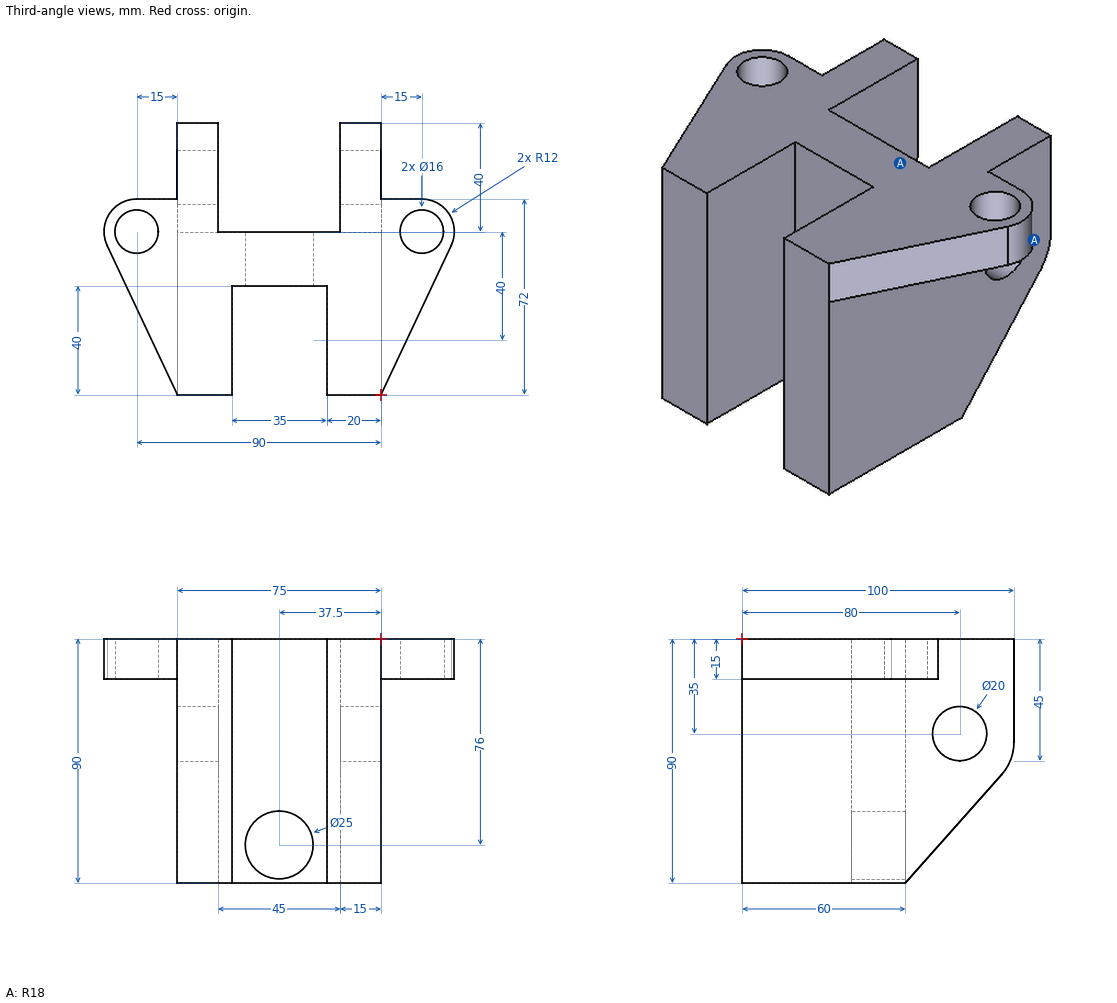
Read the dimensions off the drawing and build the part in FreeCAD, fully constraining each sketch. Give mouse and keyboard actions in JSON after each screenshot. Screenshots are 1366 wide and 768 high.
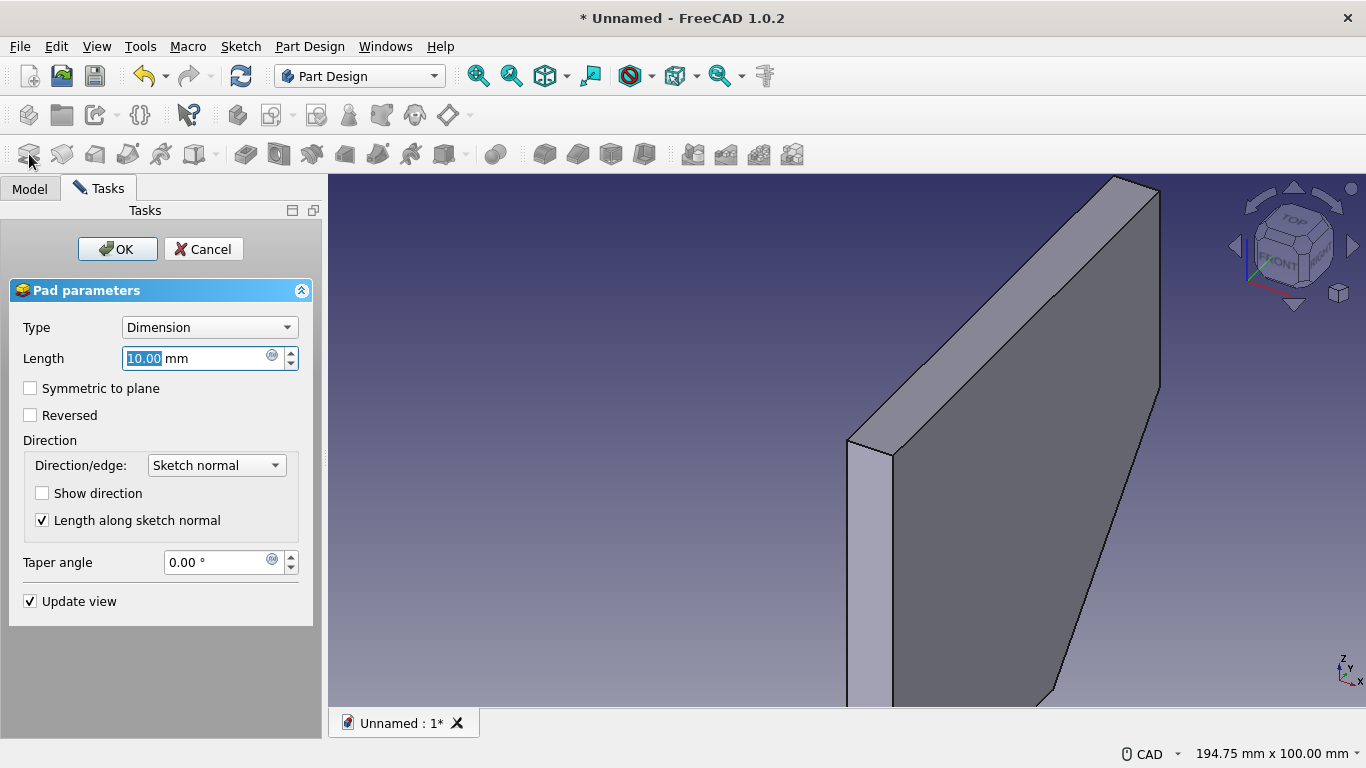
{"action": "type", "text": "75"}
{"action": "key", "text": "Tab"}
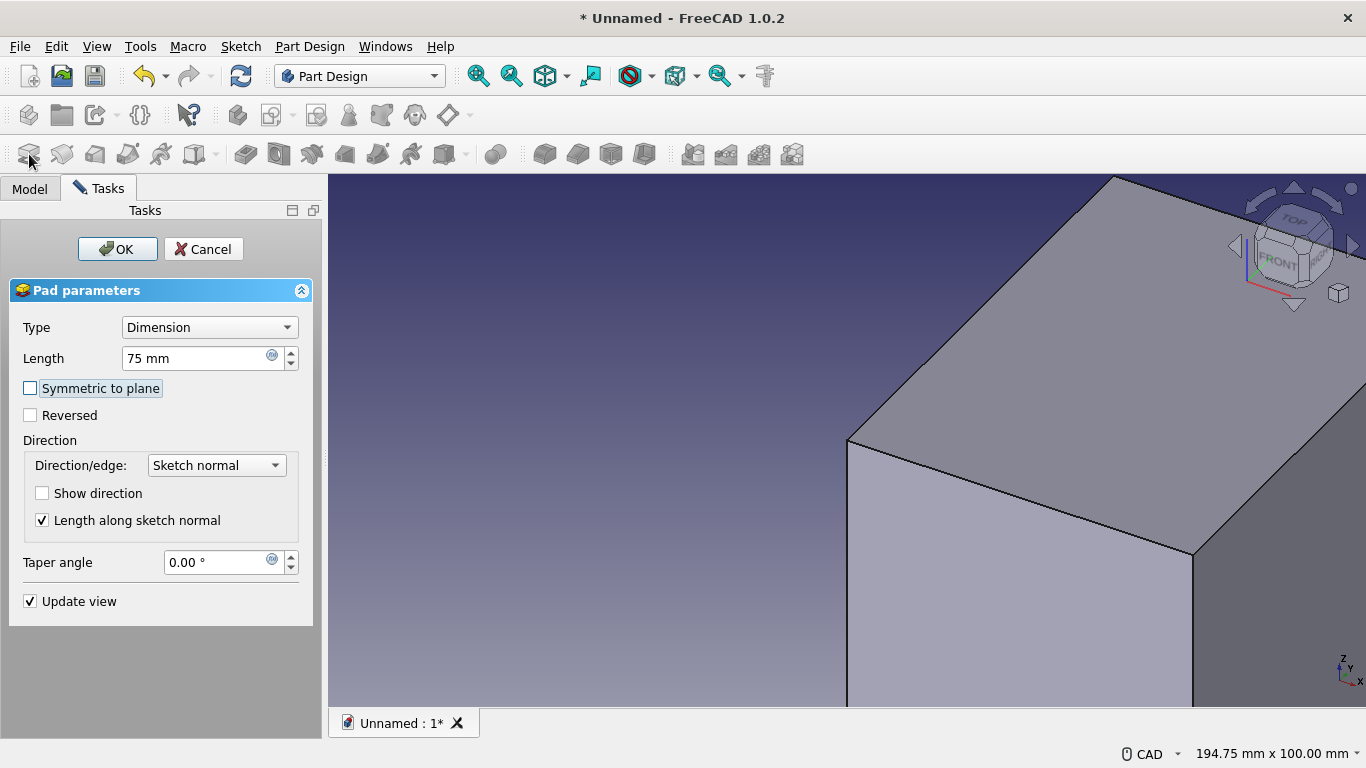
{"action": "left_click", "coordinate": [31, 415]}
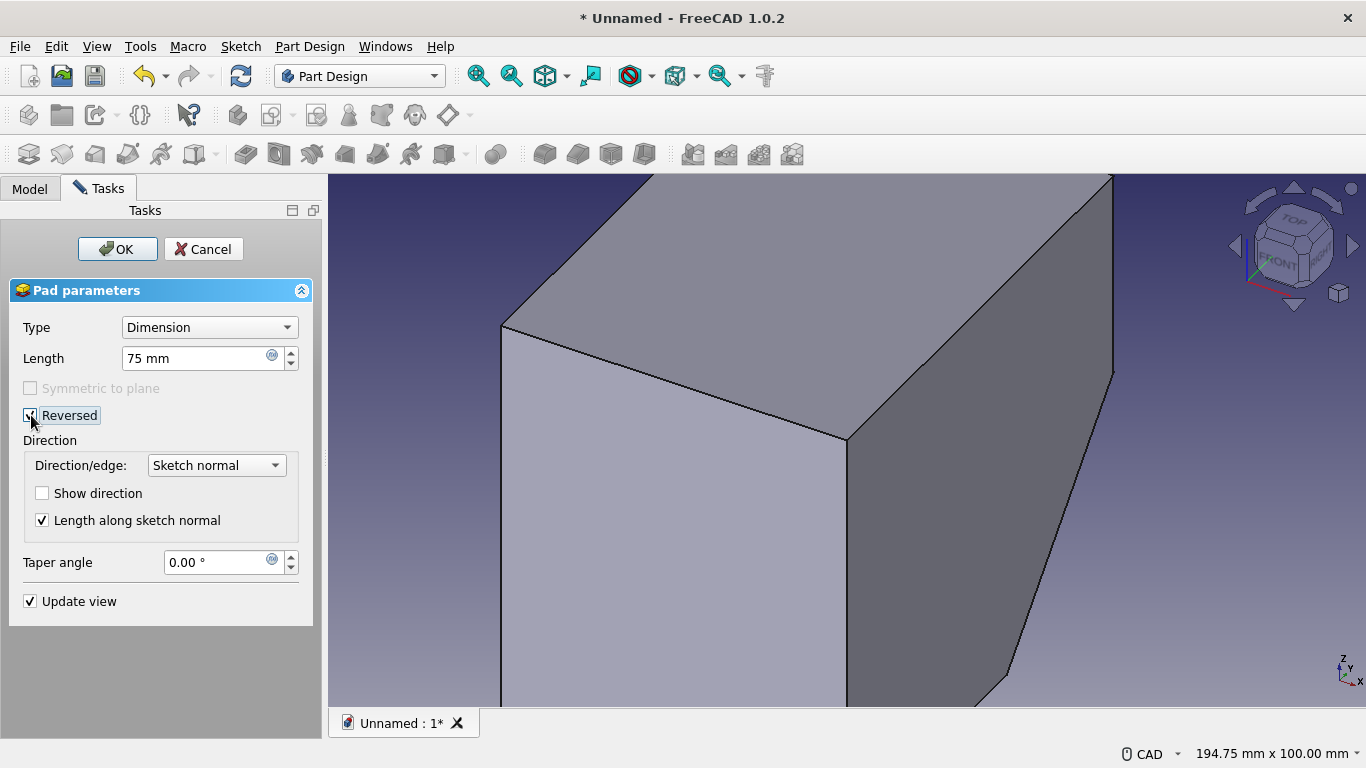
{"action": "left_click", "coordinate": [118, 249]}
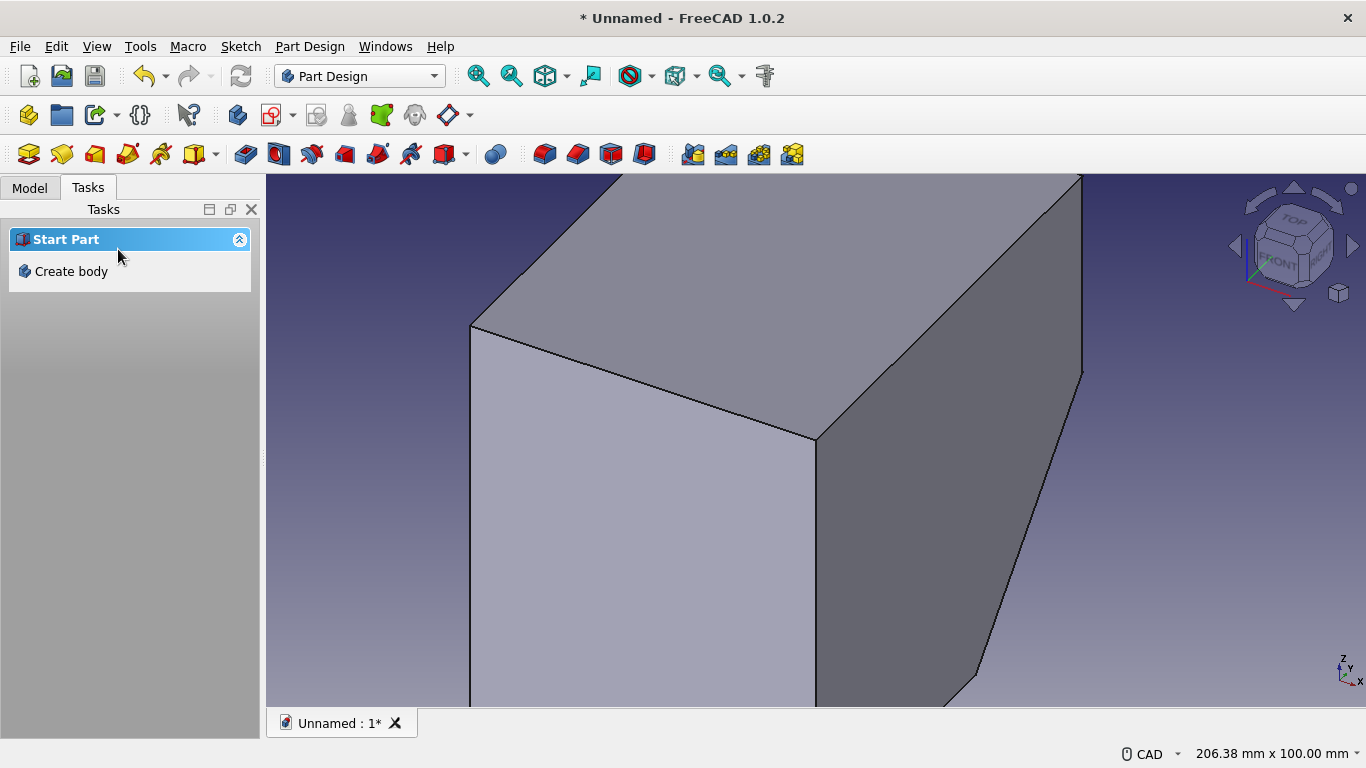
{"action": "left_click", "coordinate": [479, 76]}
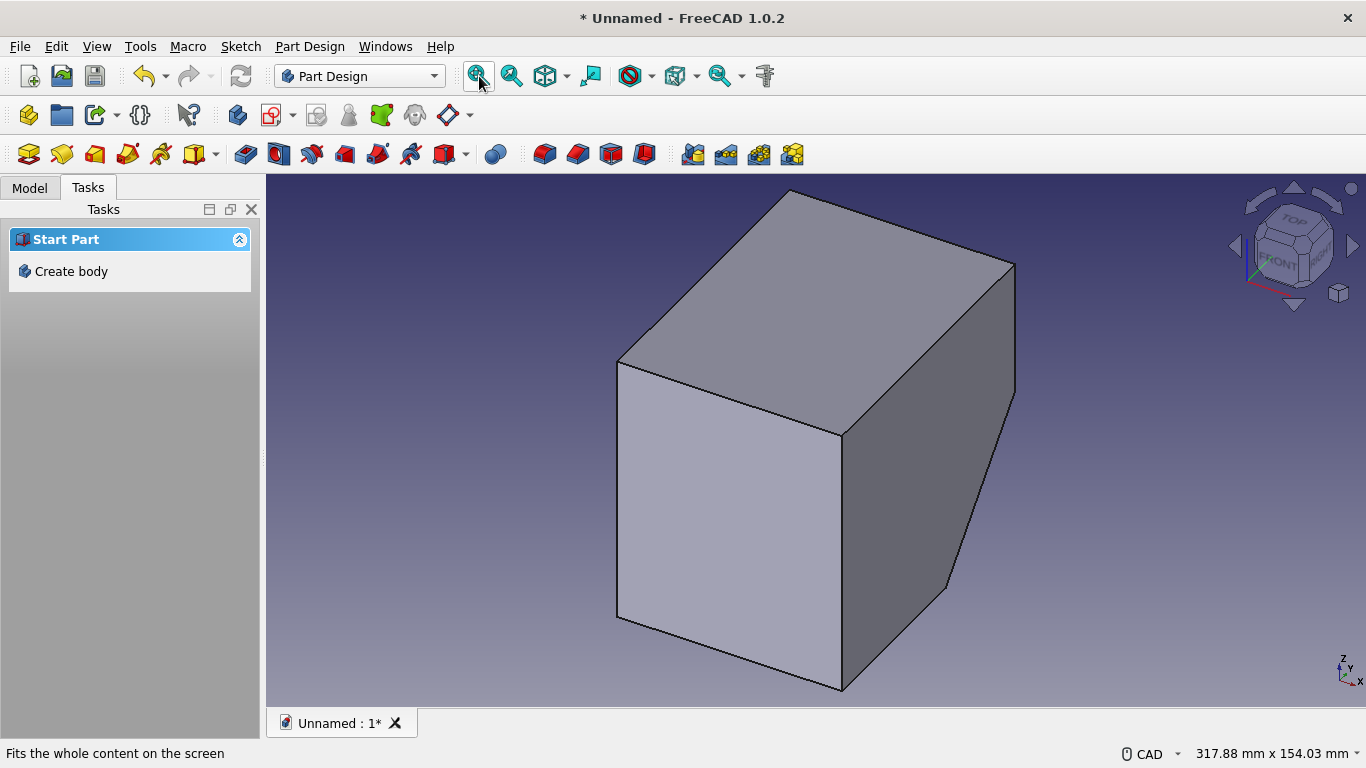
{"action": "key", "text": "5"}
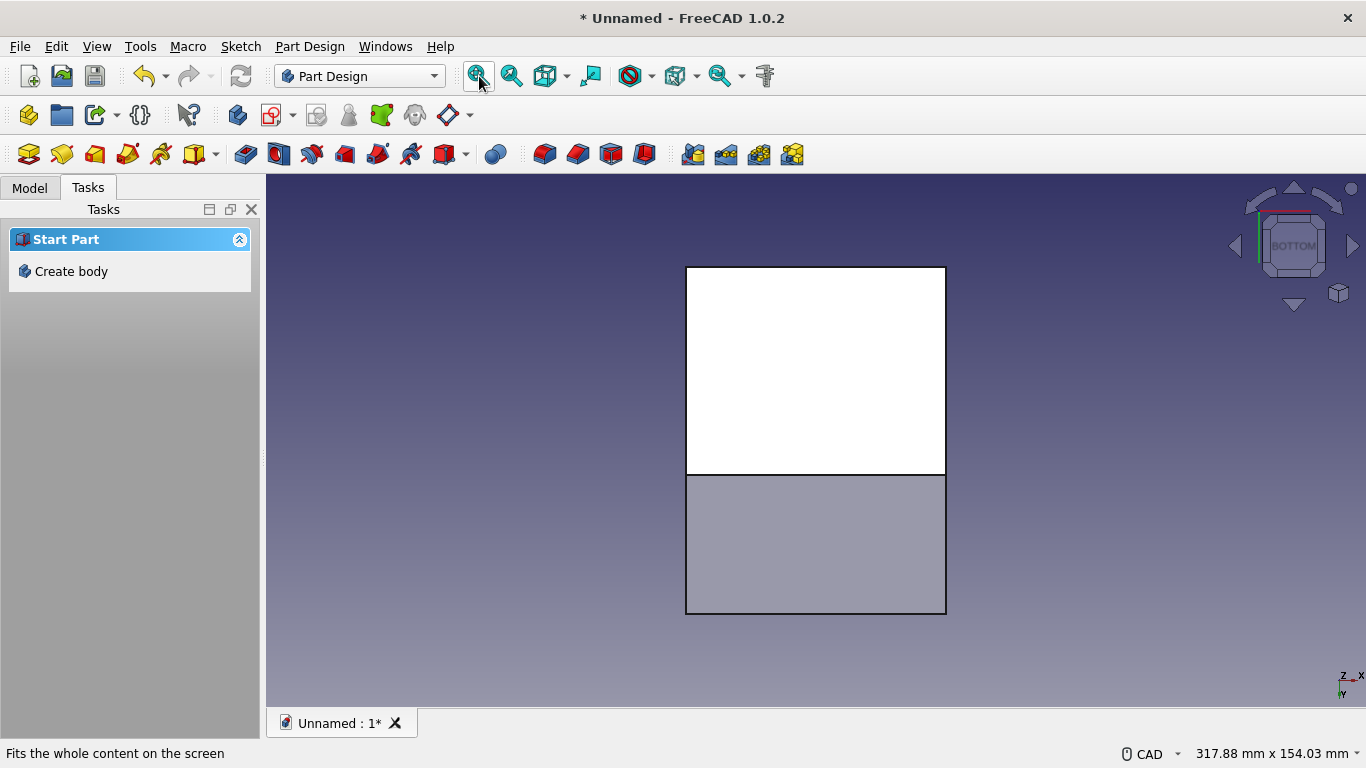
{"action": "left_click", "coordinate": [816, 370]}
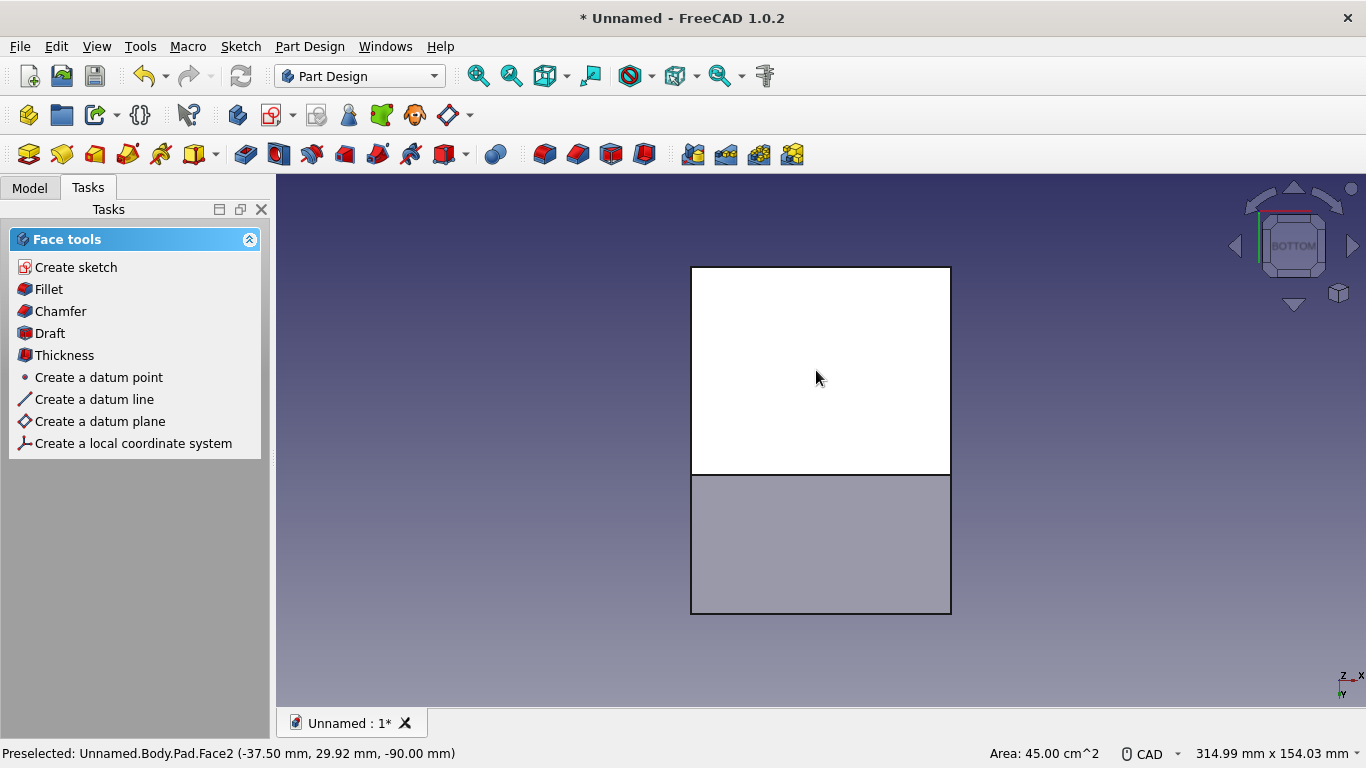
{"action": "left_click", "coordinate": [270, 116]}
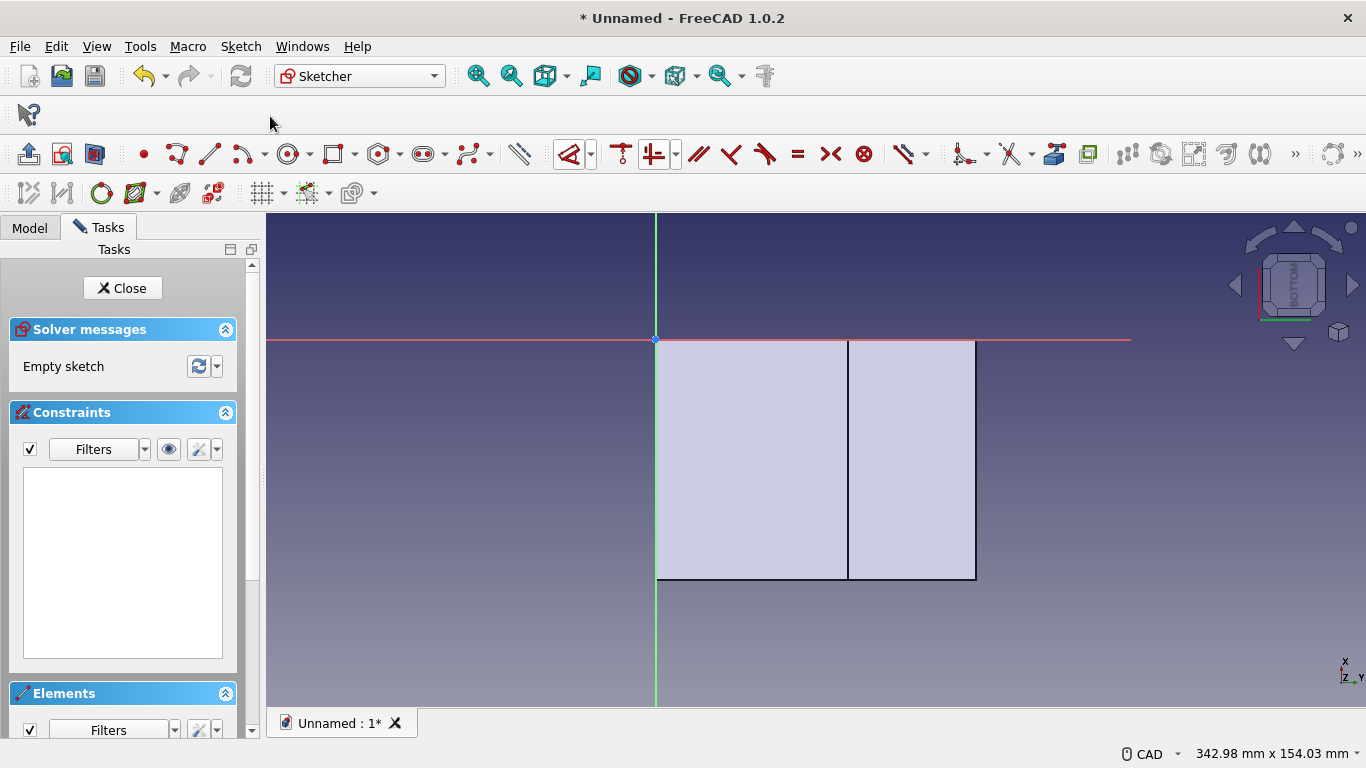
{"action": "scroll", "coordinate": [686, 389], "scroll_direction": "up", "scroll_amount": 3}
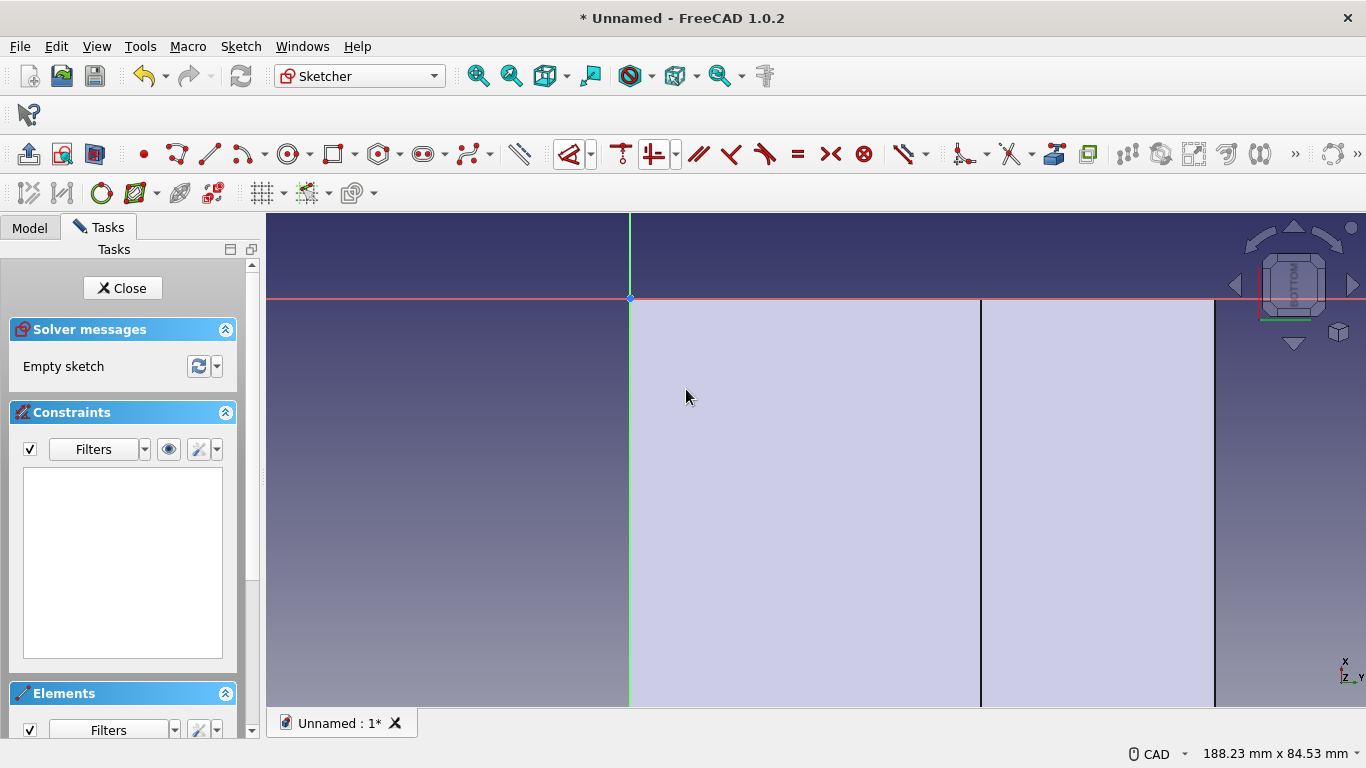
{"action": "left_click", "coordinate": [332, 154]}